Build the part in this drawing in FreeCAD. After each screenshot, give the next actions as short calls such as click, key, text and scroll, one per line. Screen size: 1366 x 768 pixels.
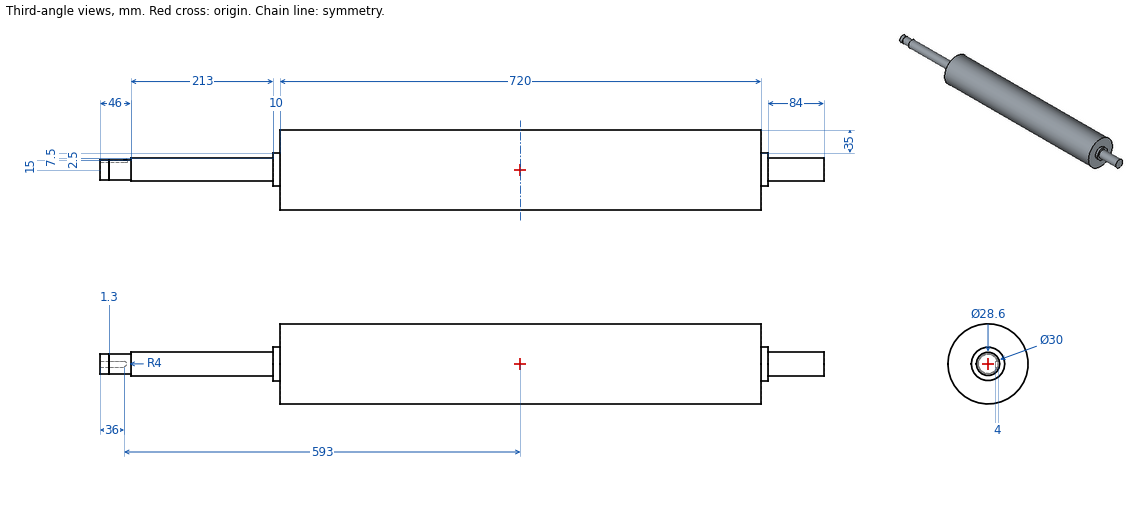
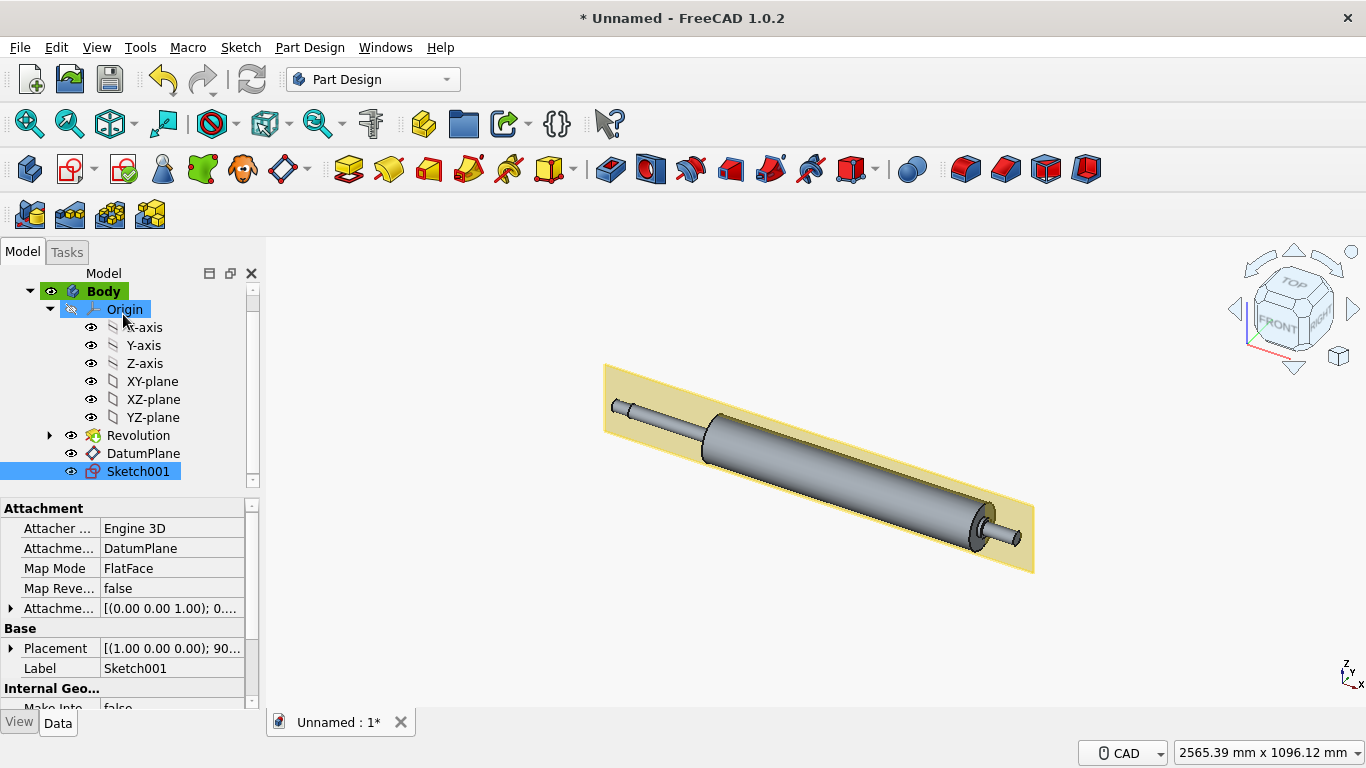
click(612, 170)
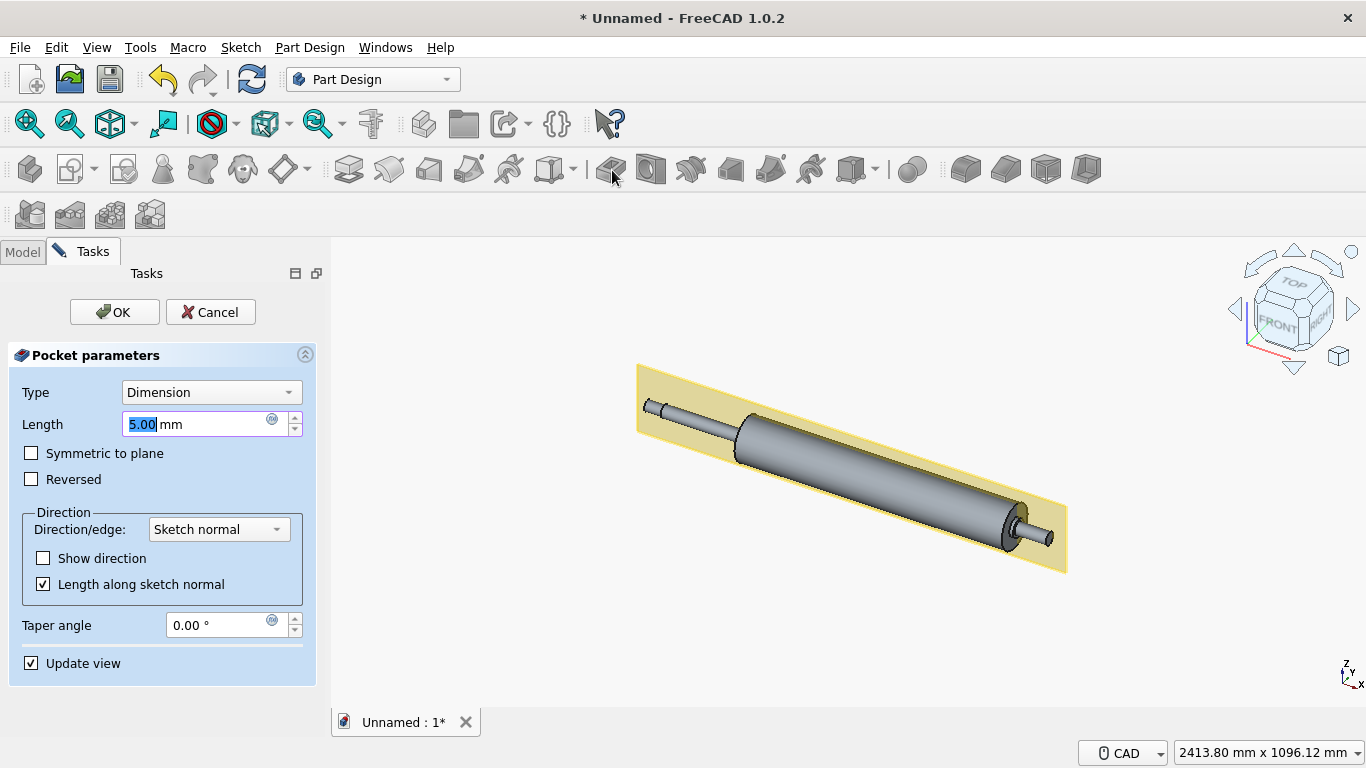
text(4)
key(Tab)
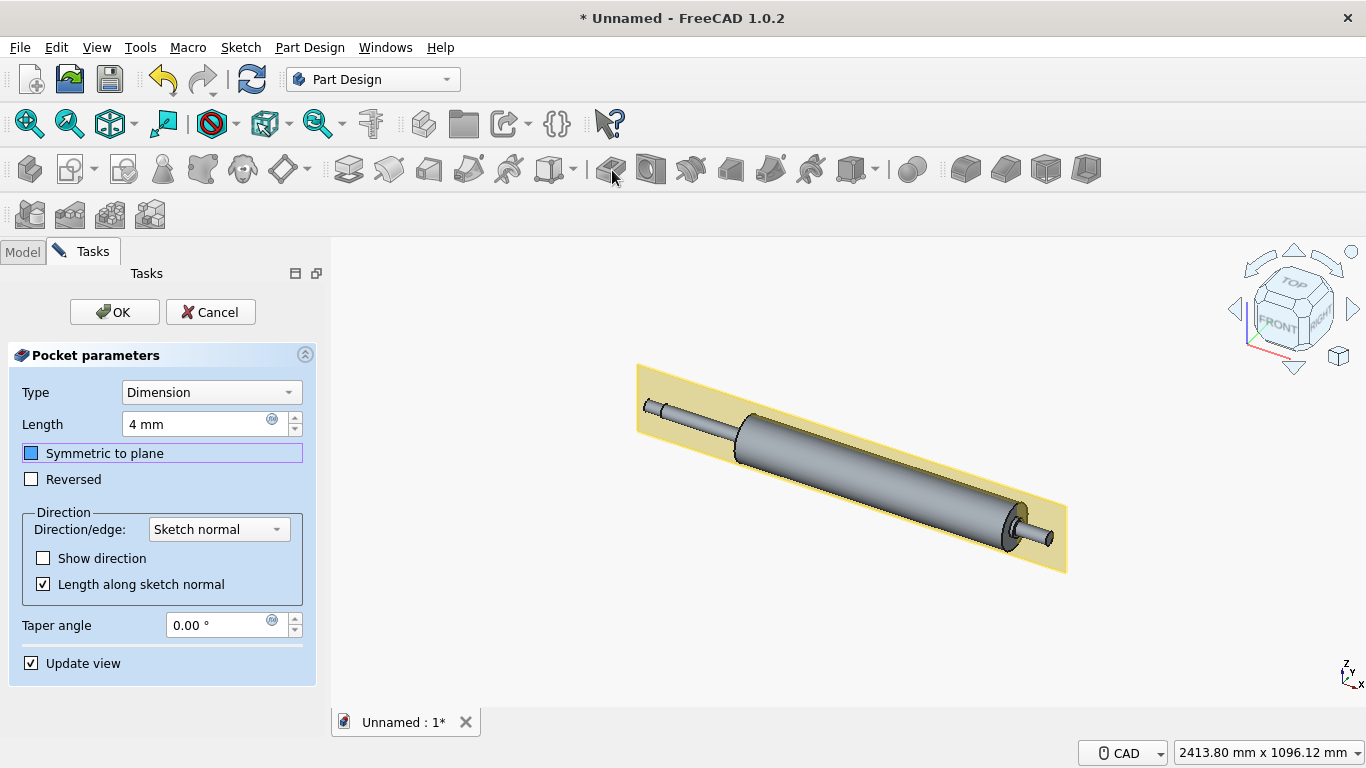
click(30, 479)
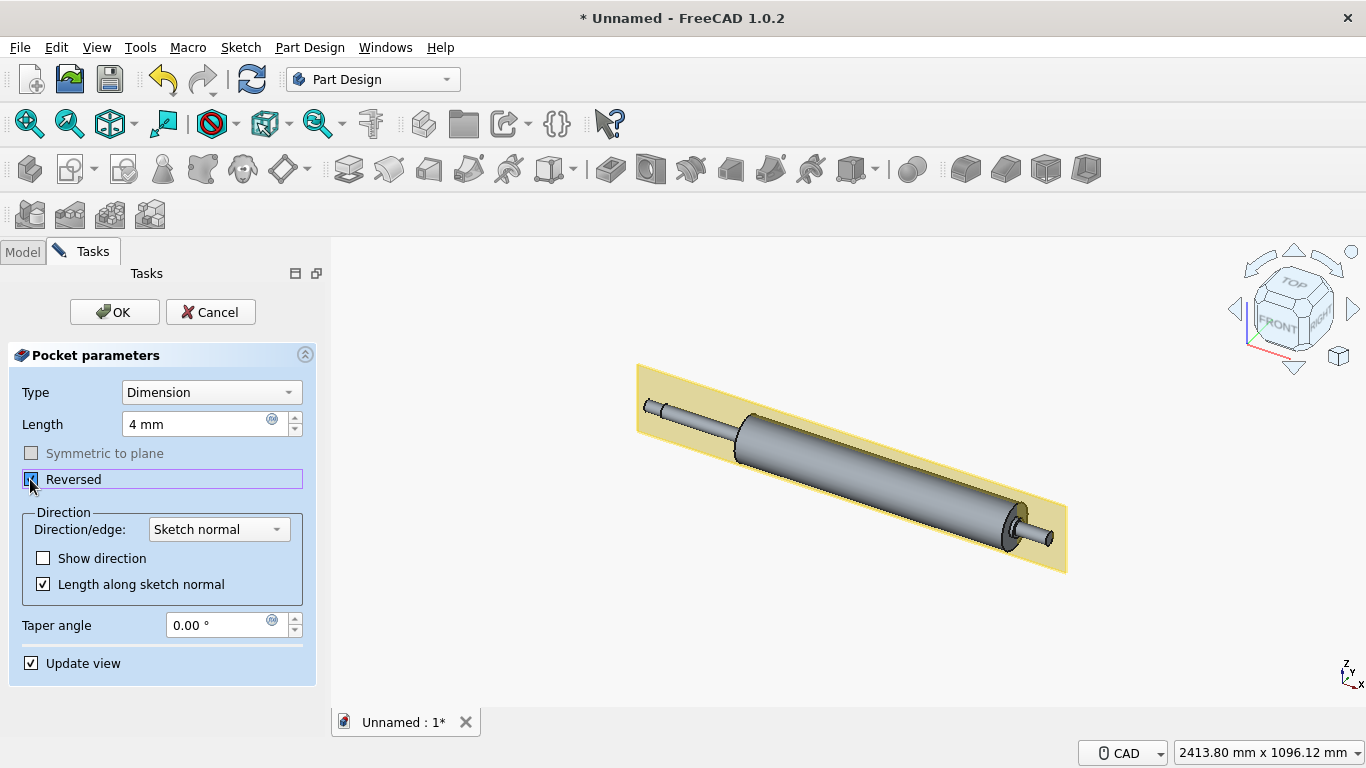
click(115, 312)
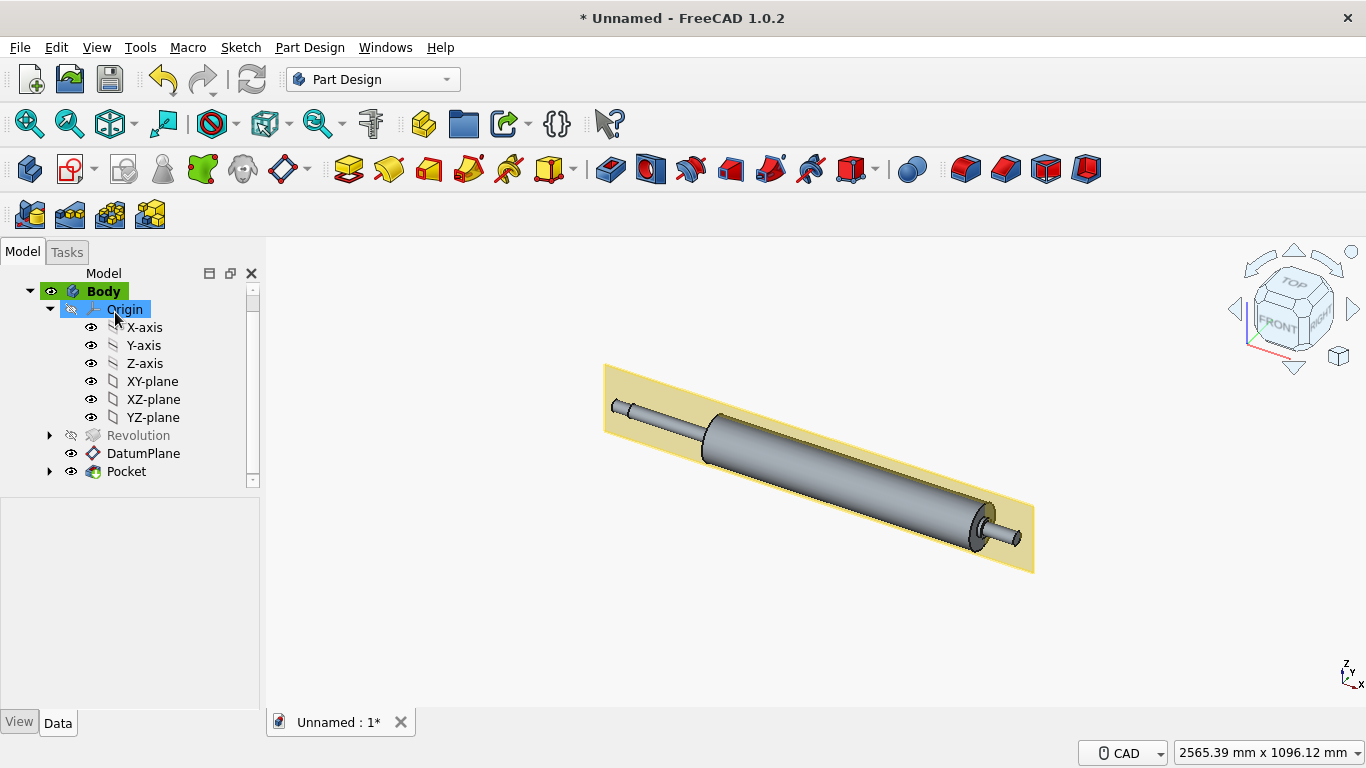
click(116, 453)
key(space)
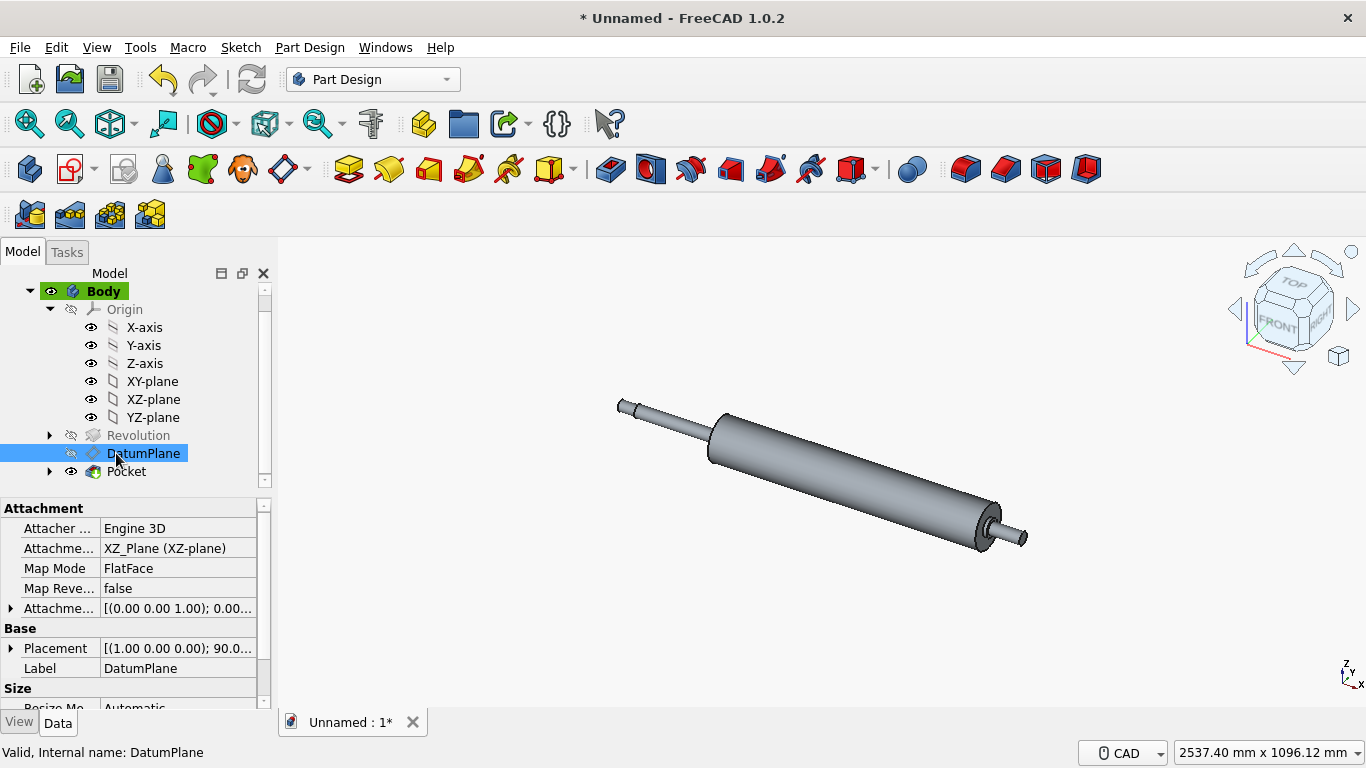
click(30, 124)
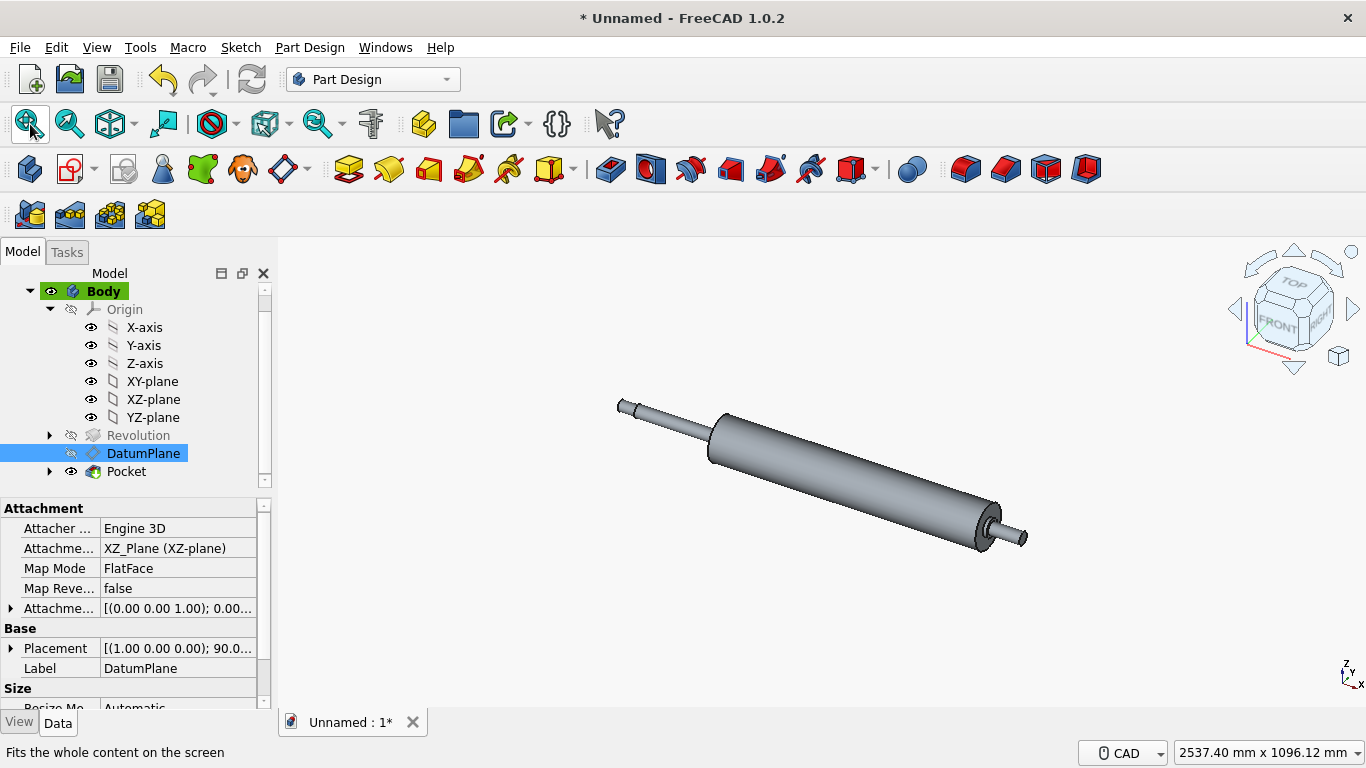
click(136, 417)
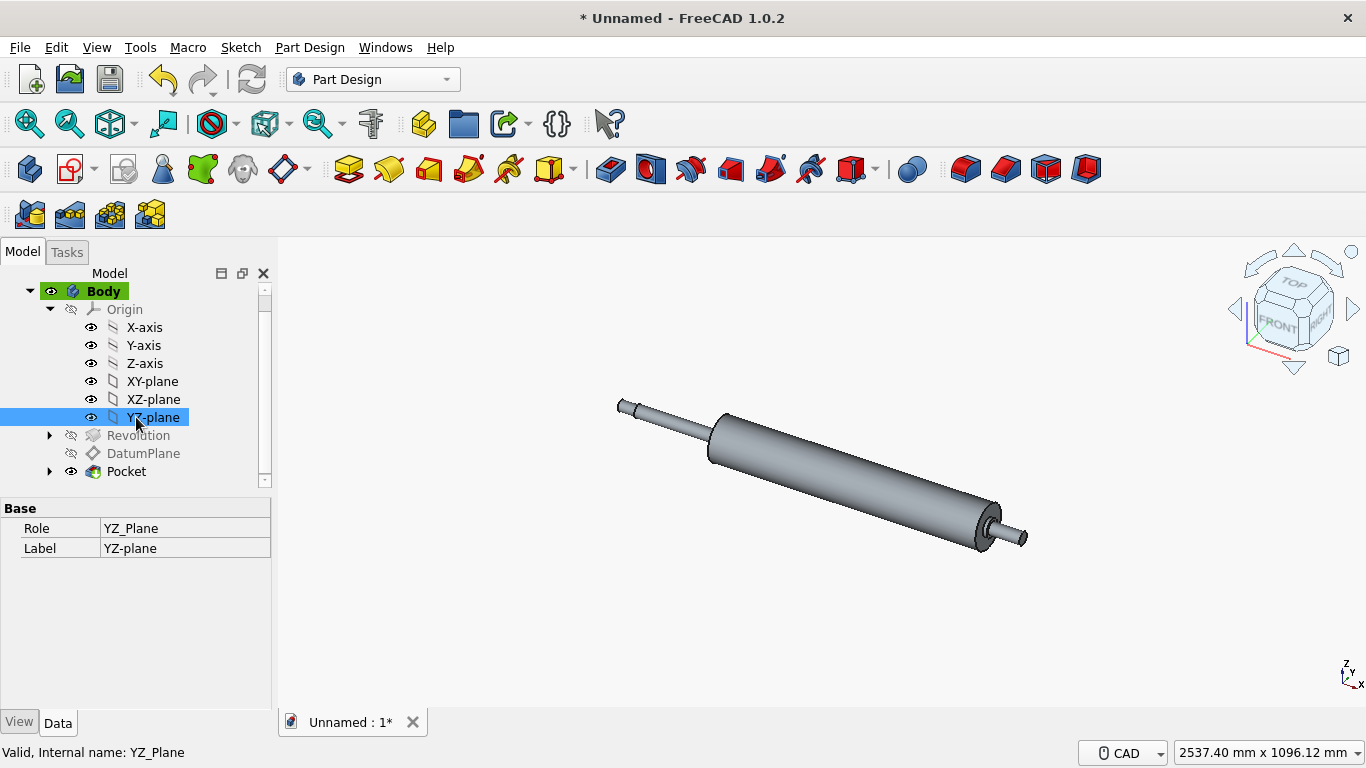
click(284, 170)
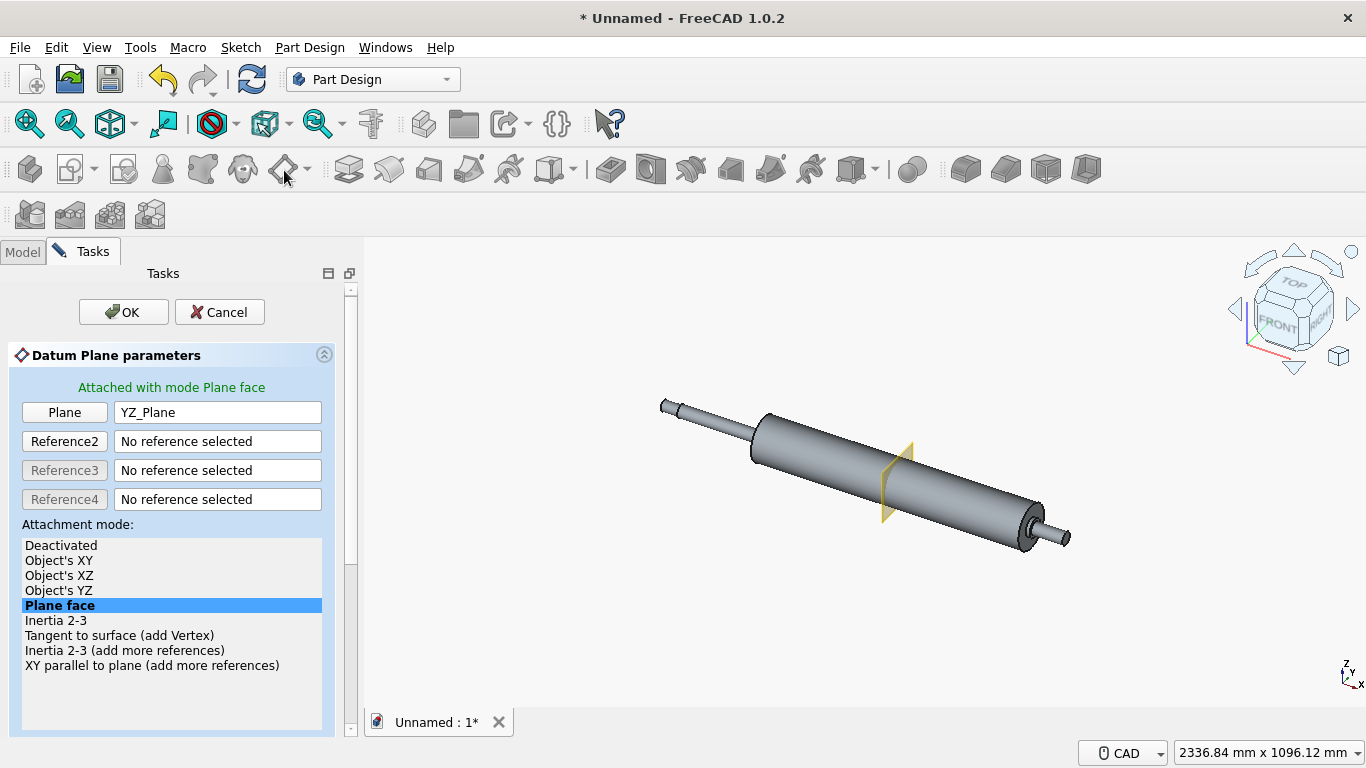
scroll(351, 510, down, 3)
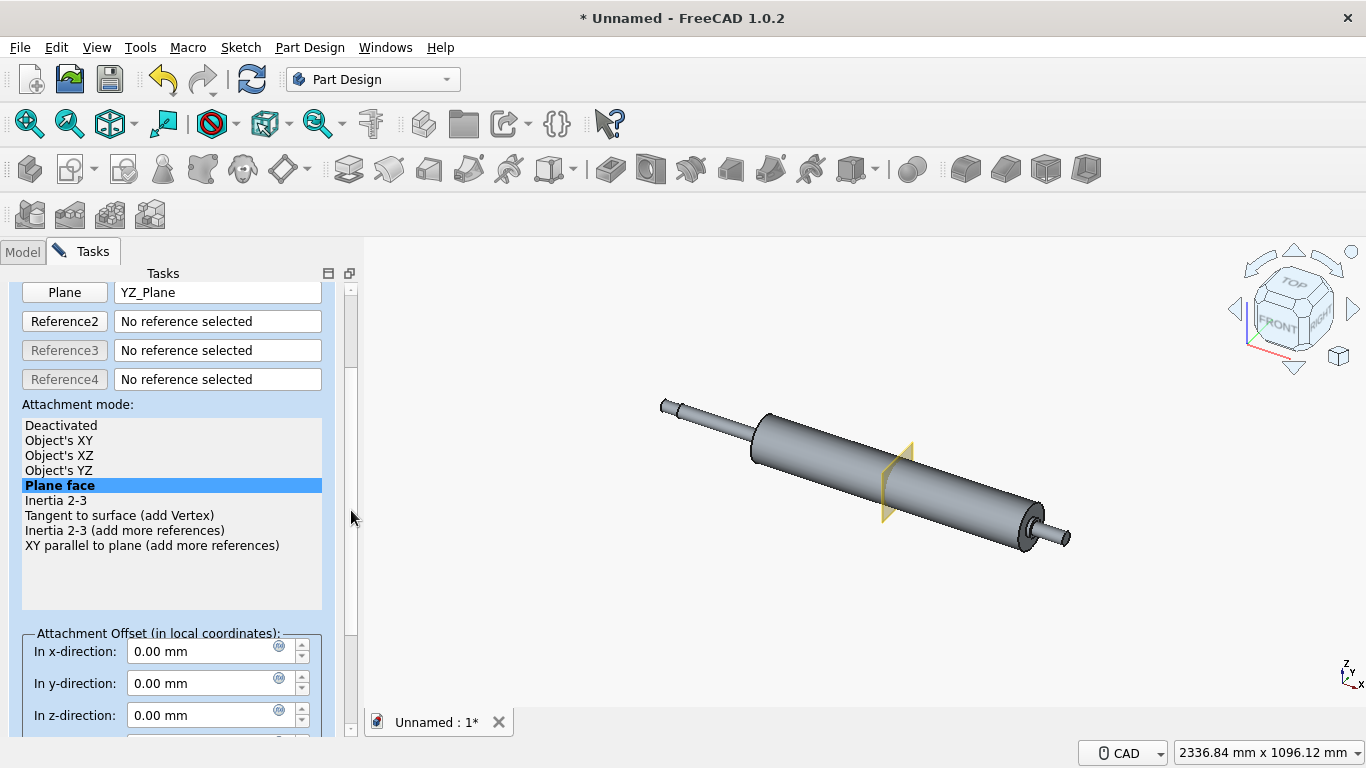
triple_click(210, 655)